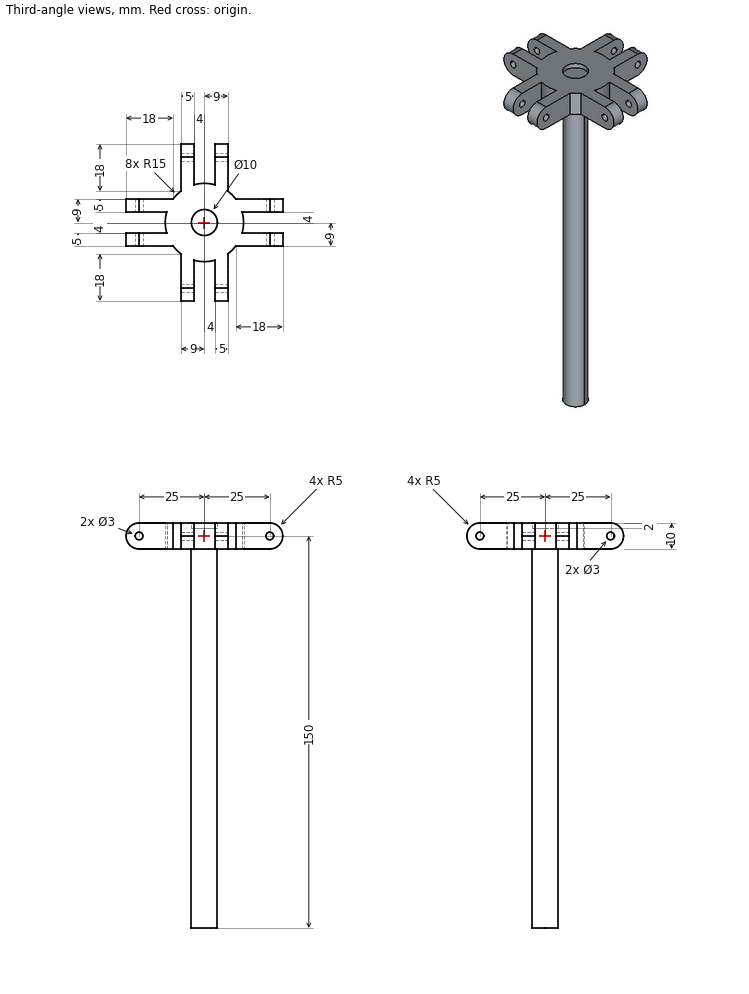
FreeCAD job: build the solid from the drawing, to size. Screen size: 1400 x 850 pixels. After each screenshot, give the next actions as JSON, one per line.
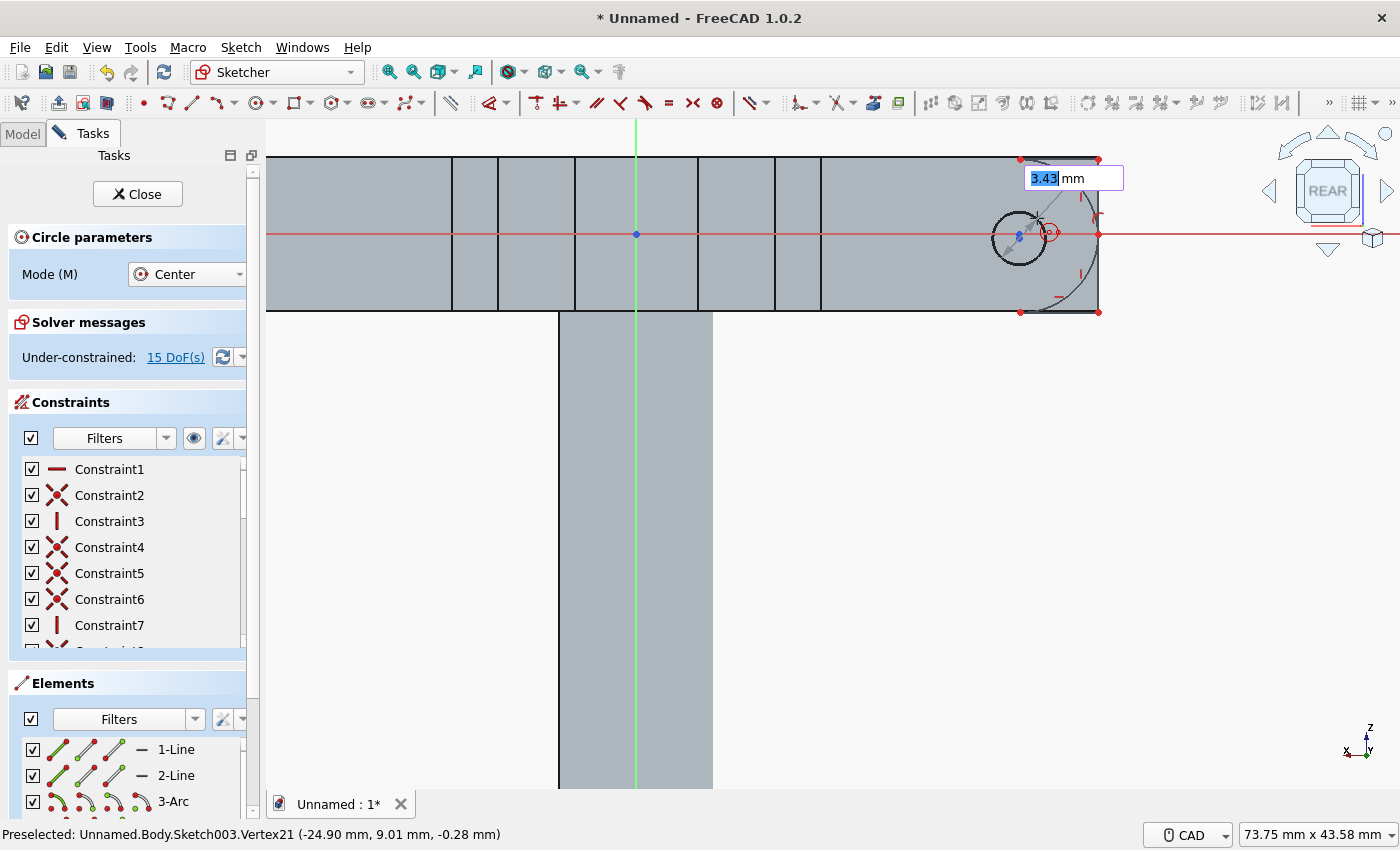
{"action": "type", "text": "3"}
{"action": "key", "text": "Return"}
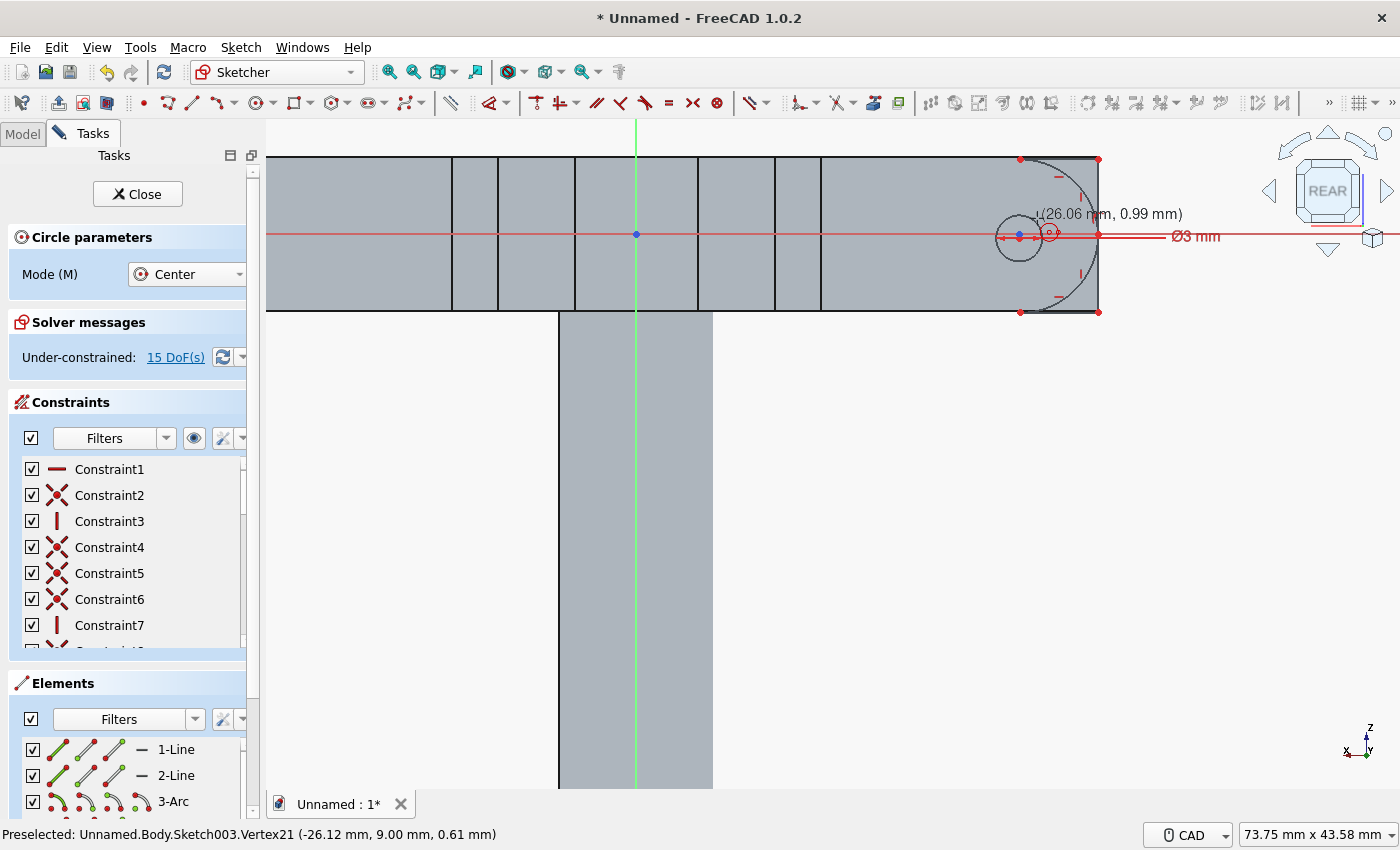
{"action": "scroll", "coordinate": [1025, 761], "scroll_direction": "down", "scroll_amount": 2}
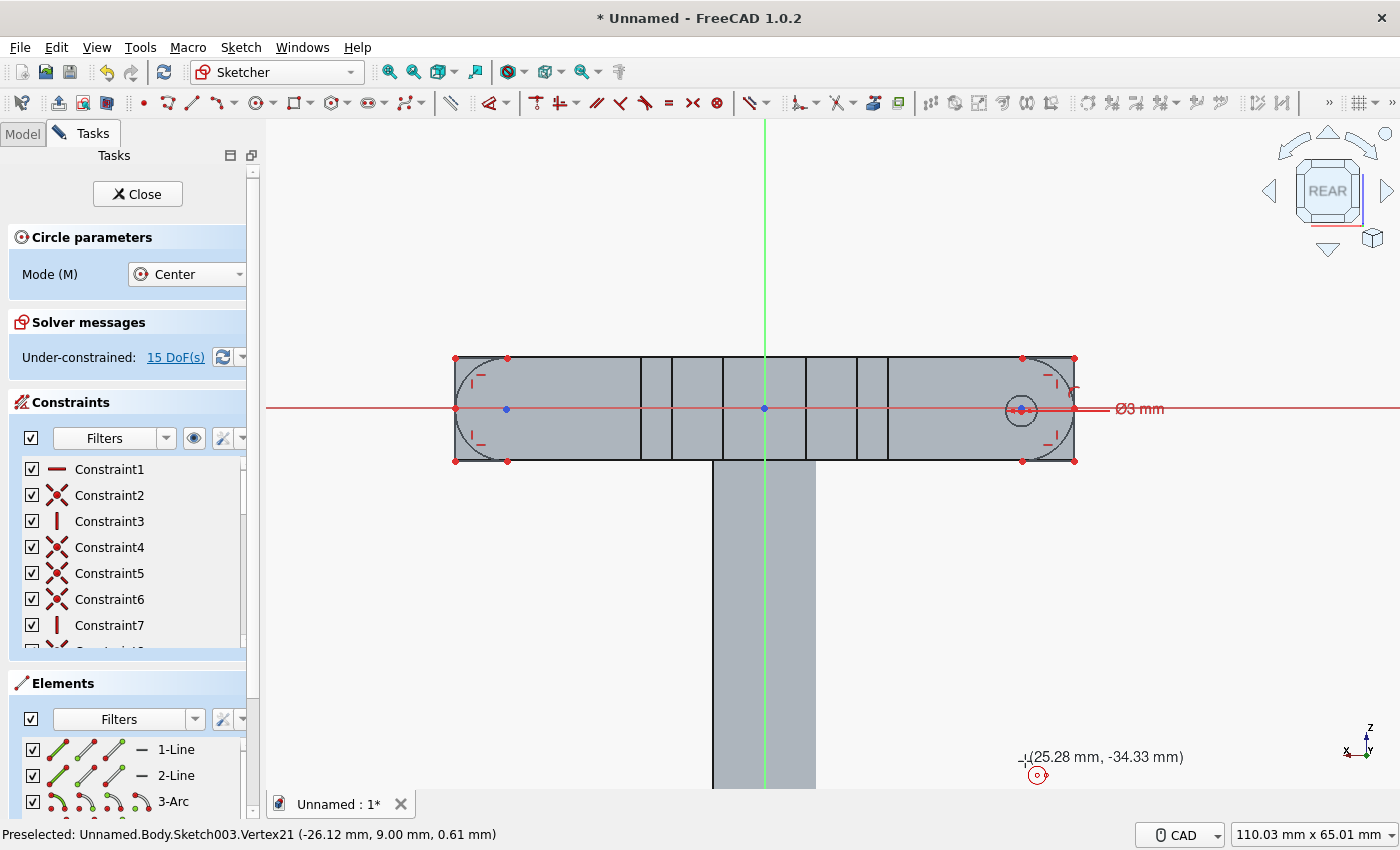
{"action": "scroll", "coordinate": [507, 408], "scroll_direction": "up", "scroll_amount": 2}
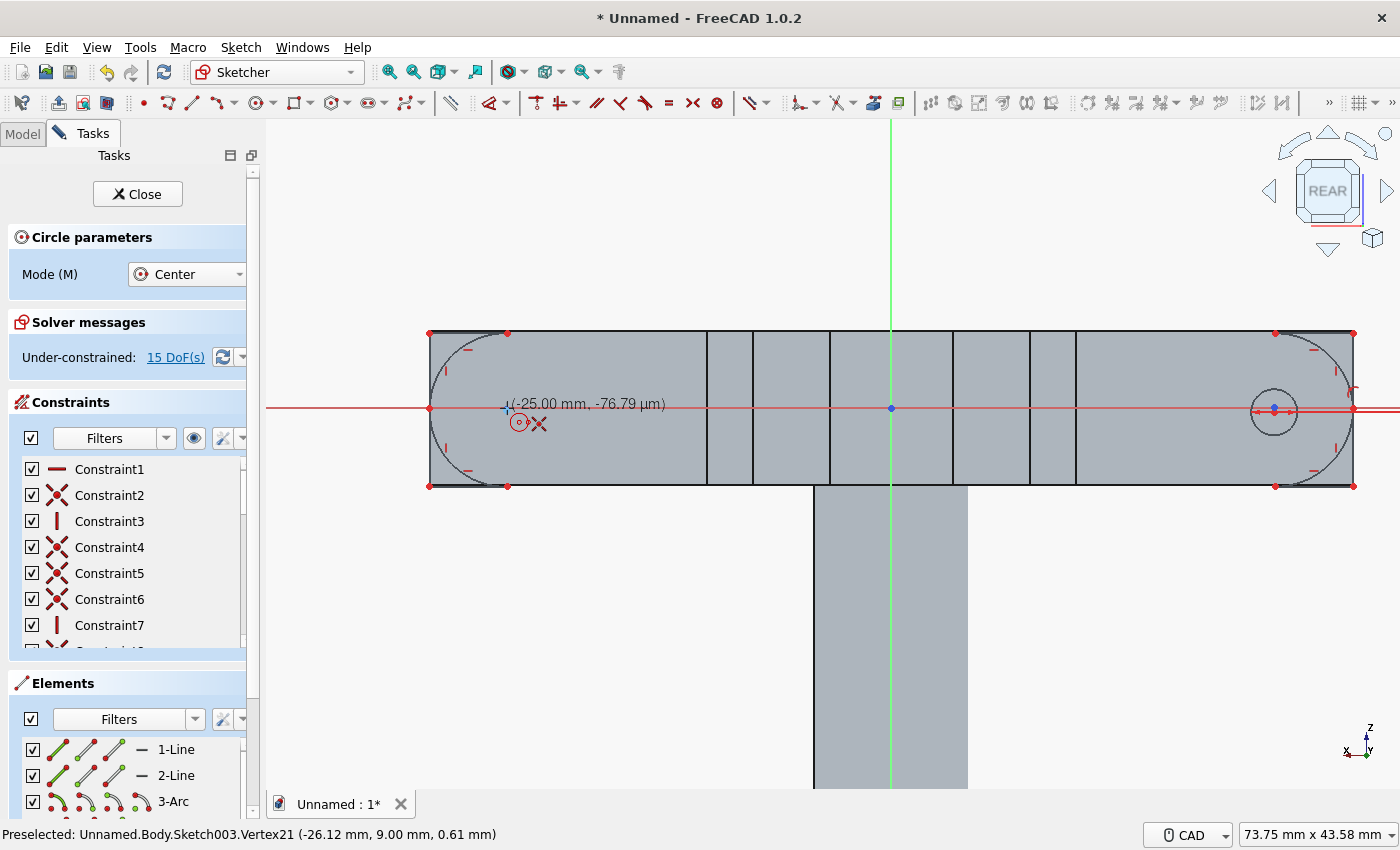
{"action": "left_click", "coordinate": [507, 408]}
{"action": "mouse_move", "coordinate": [523, 392]}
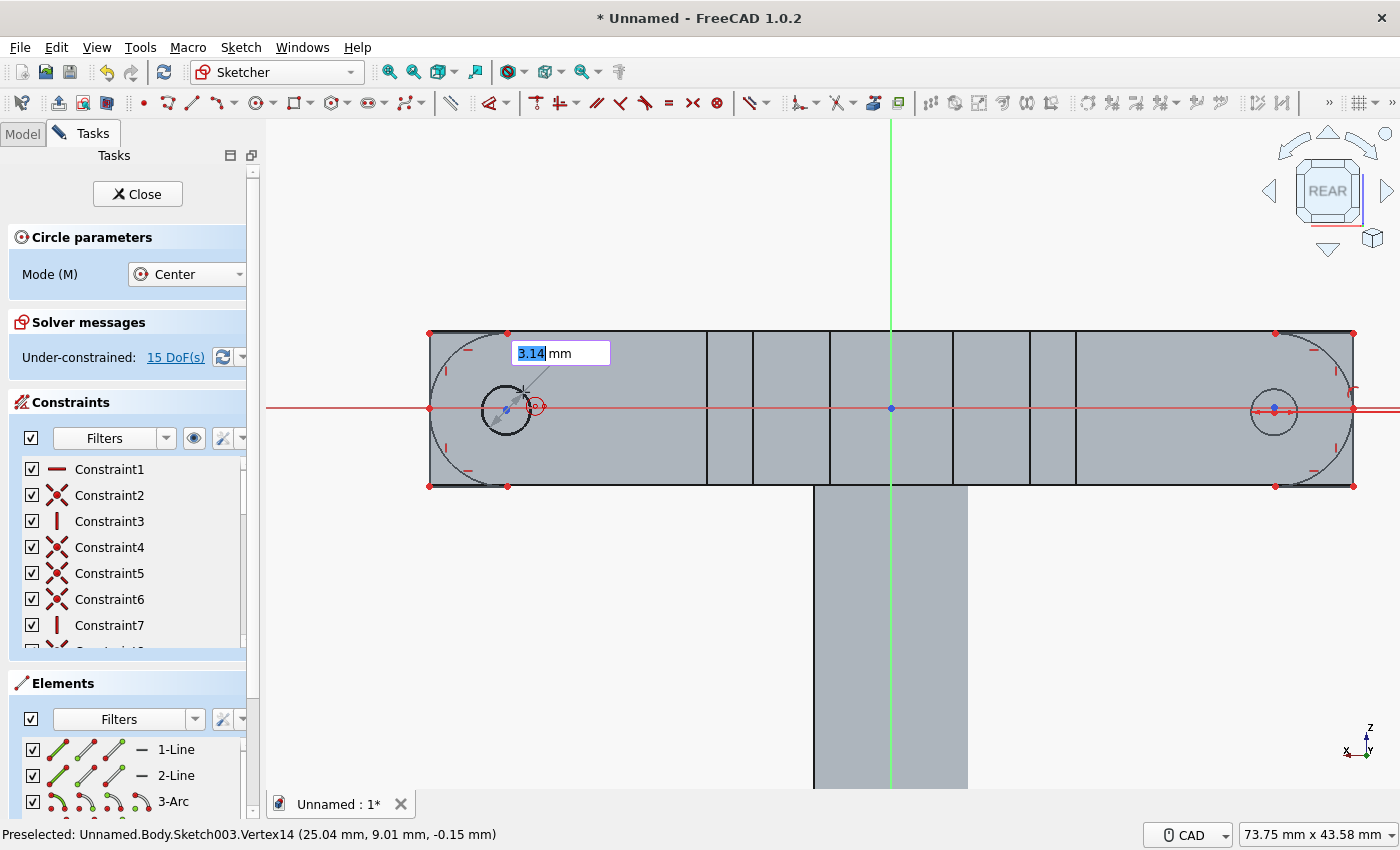
{"action": "type", "text": "3"}
{"action": "key", "text": "Return"}
{"action": "key", "text": "Escape"}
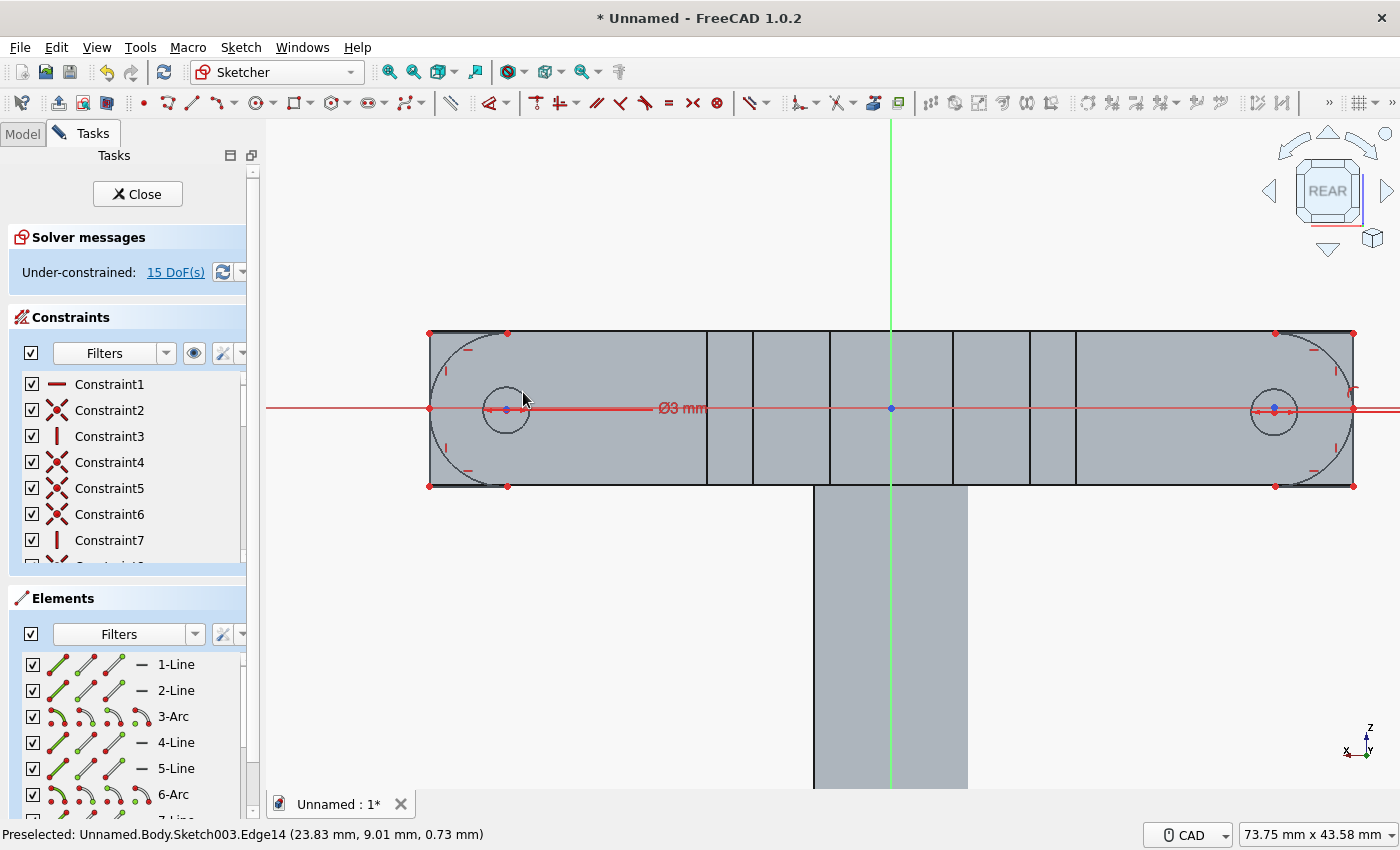
{"action": "left_click", "coordinate": [453, 333]}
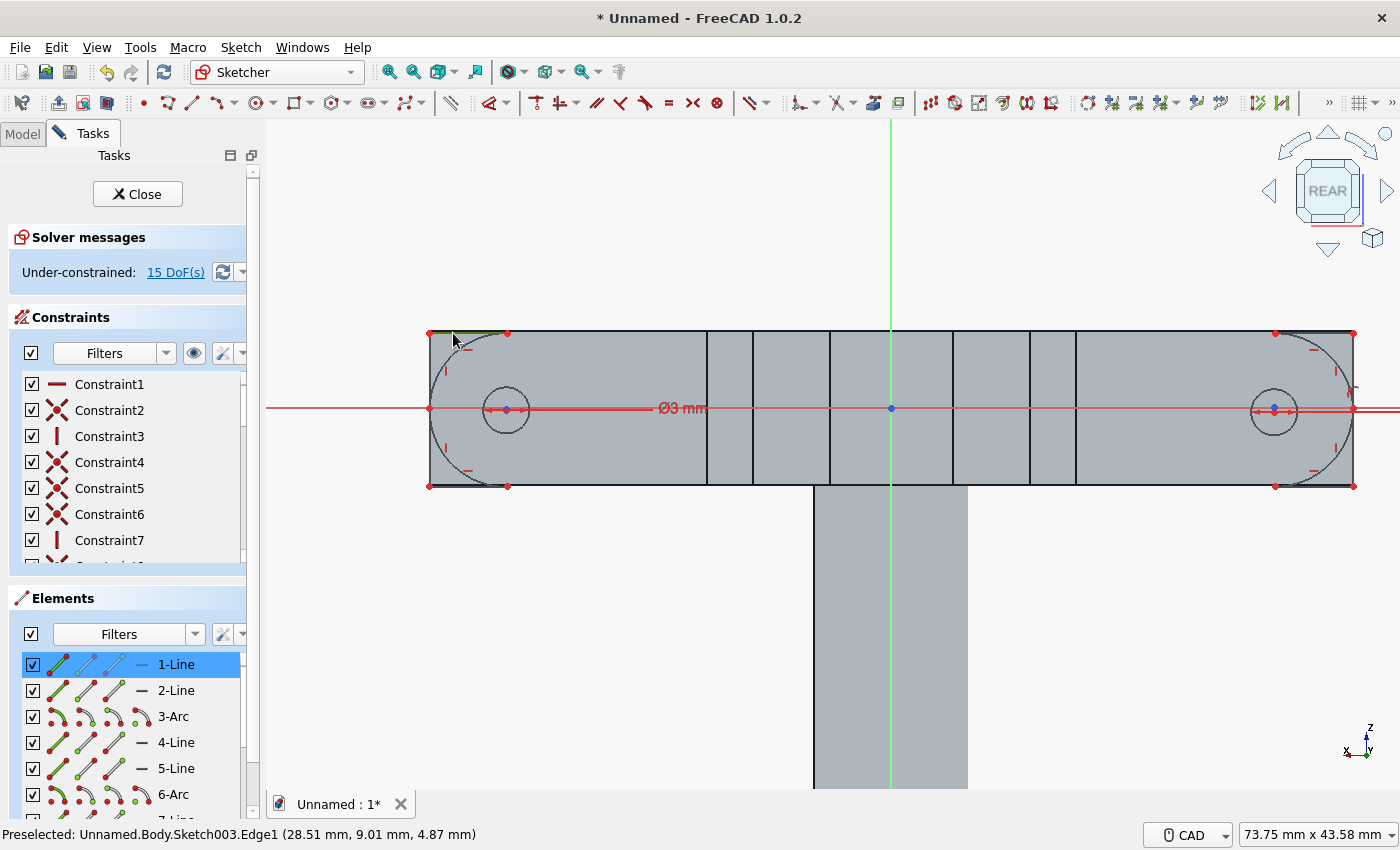
{"action": "left_click", "coordinate": [453, 355]}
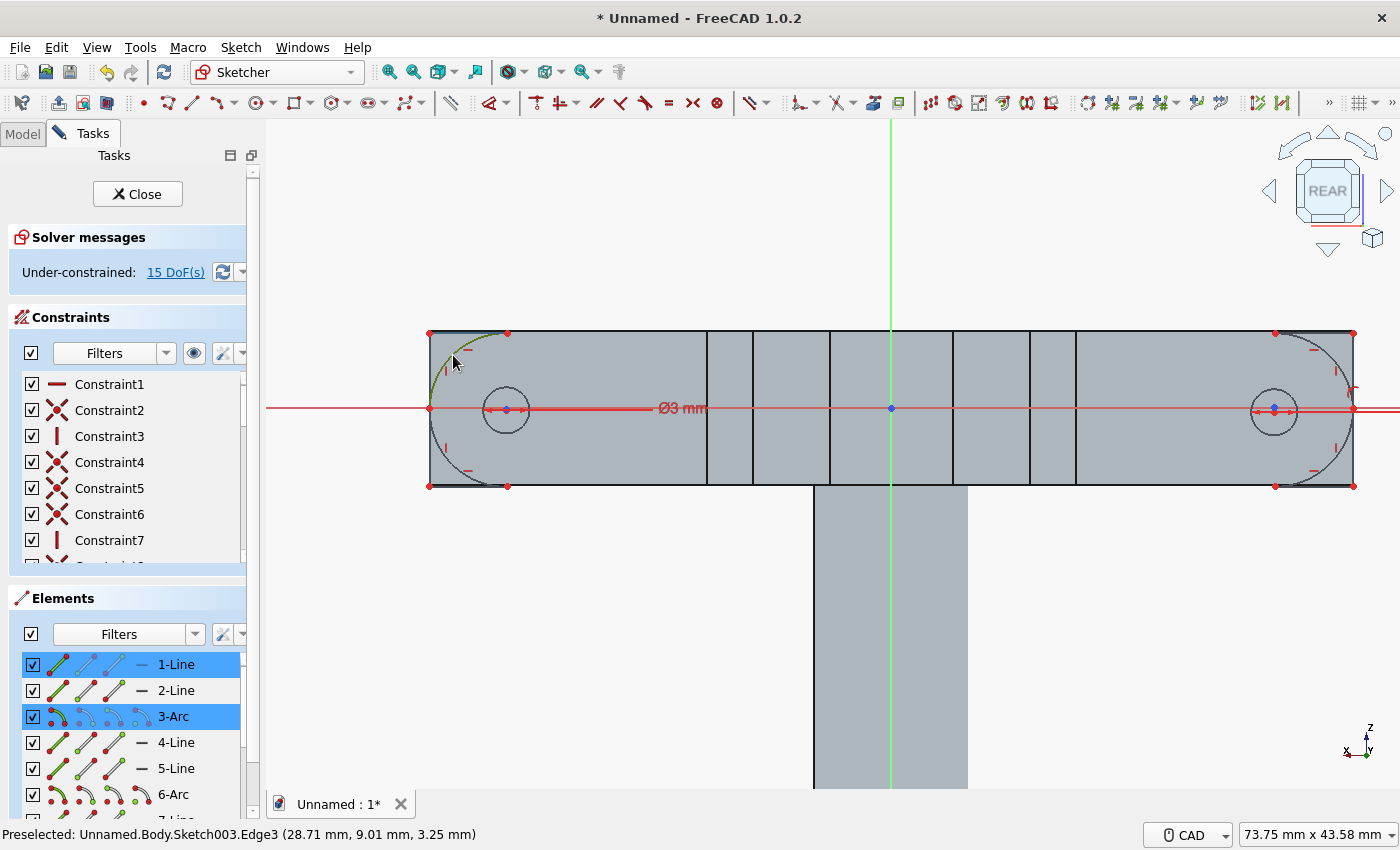
{"action": "key", "text": "t"}